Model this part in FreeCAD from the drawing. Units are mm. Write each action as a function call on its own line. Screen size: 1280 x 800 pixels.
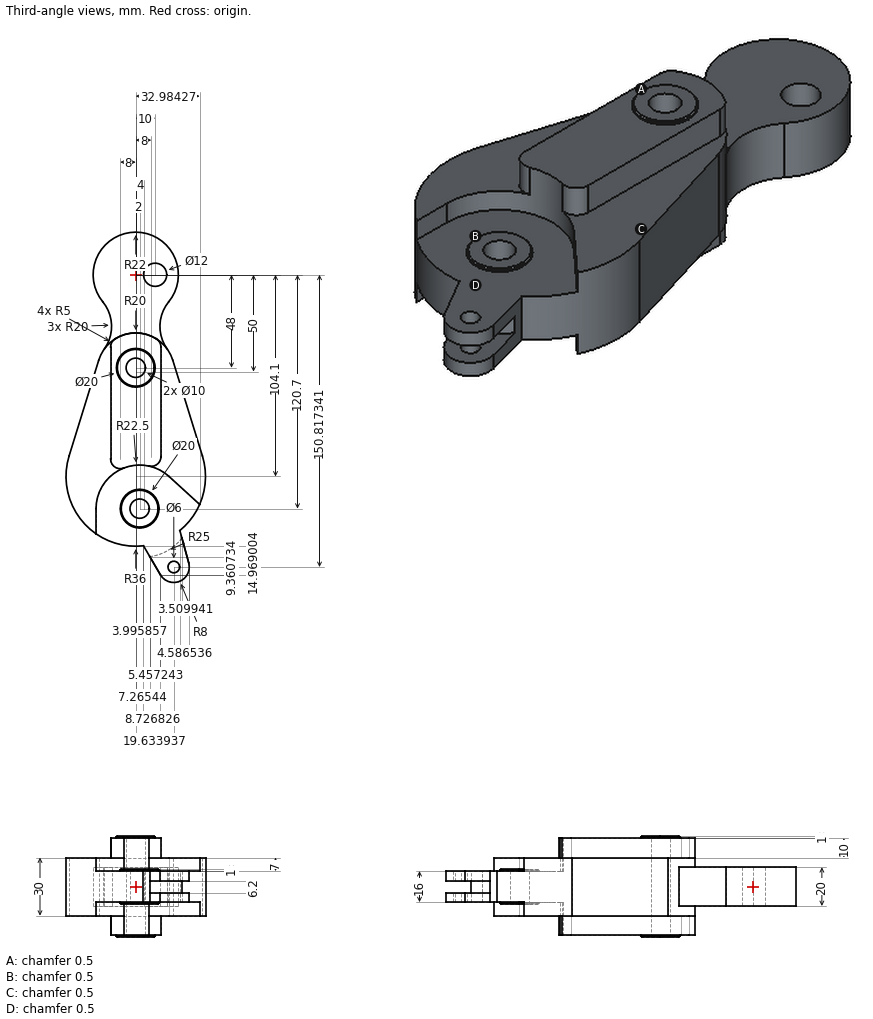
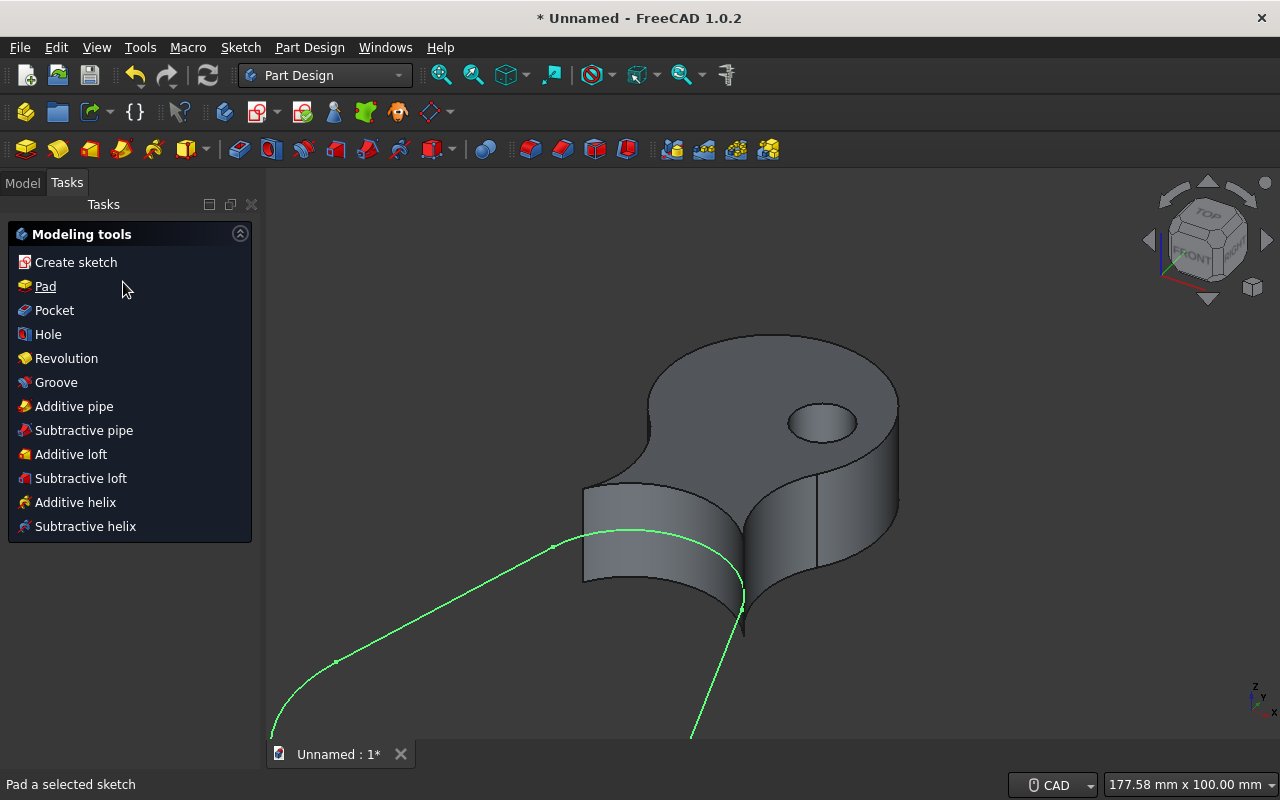
click(26, 150)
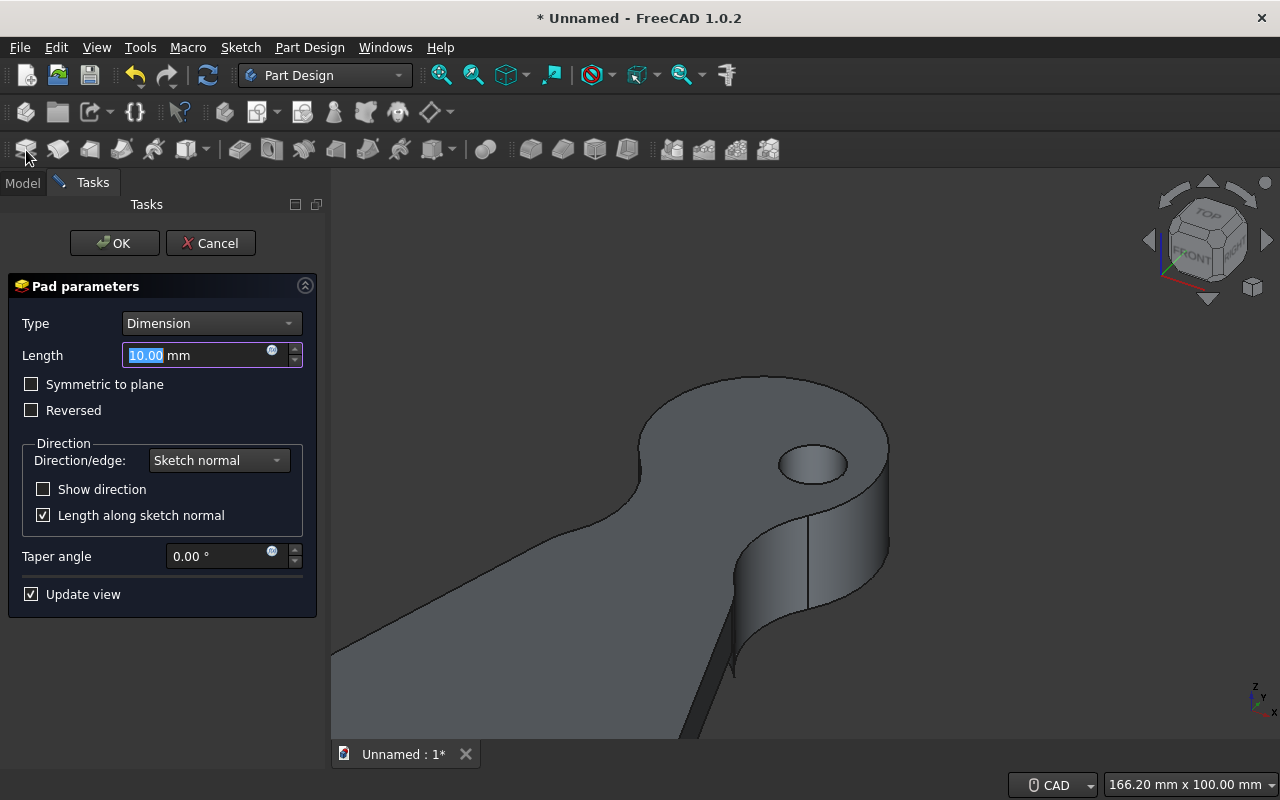
text(30)
key(Tab)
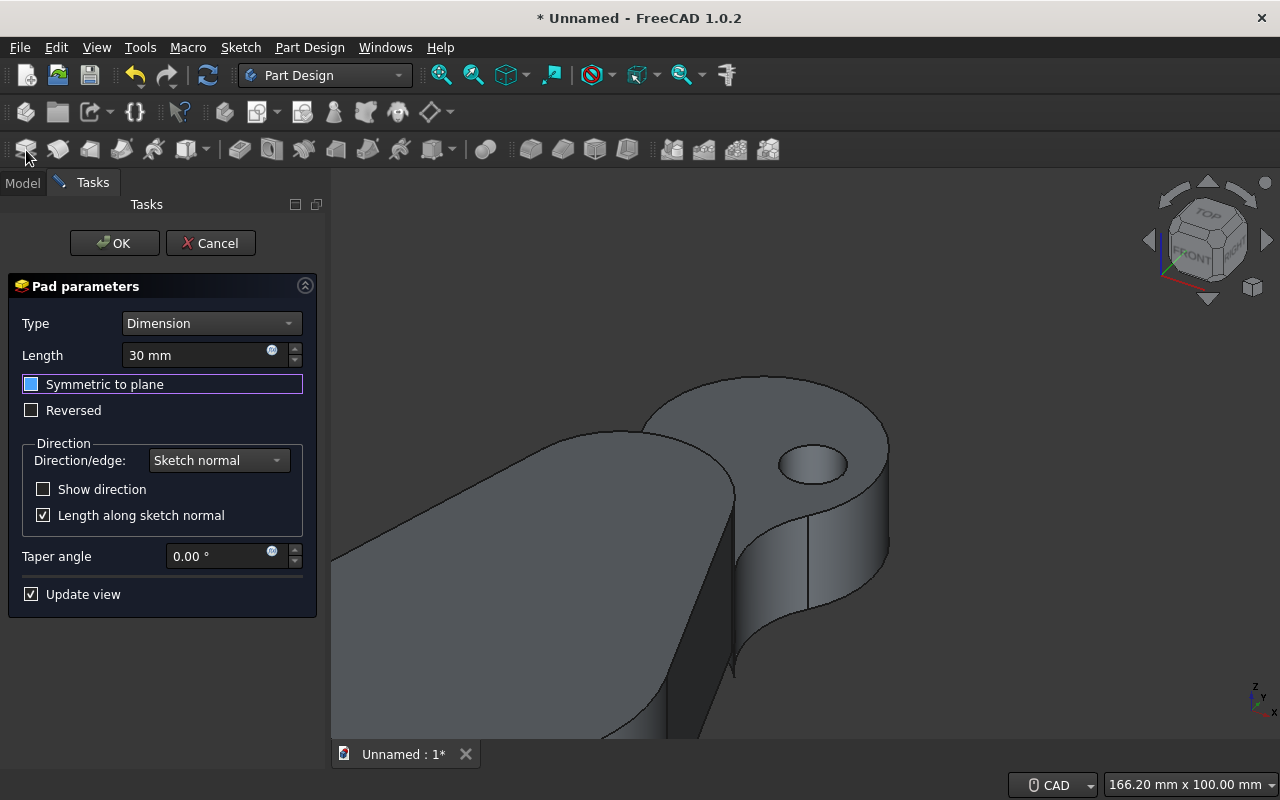
click(30, 384)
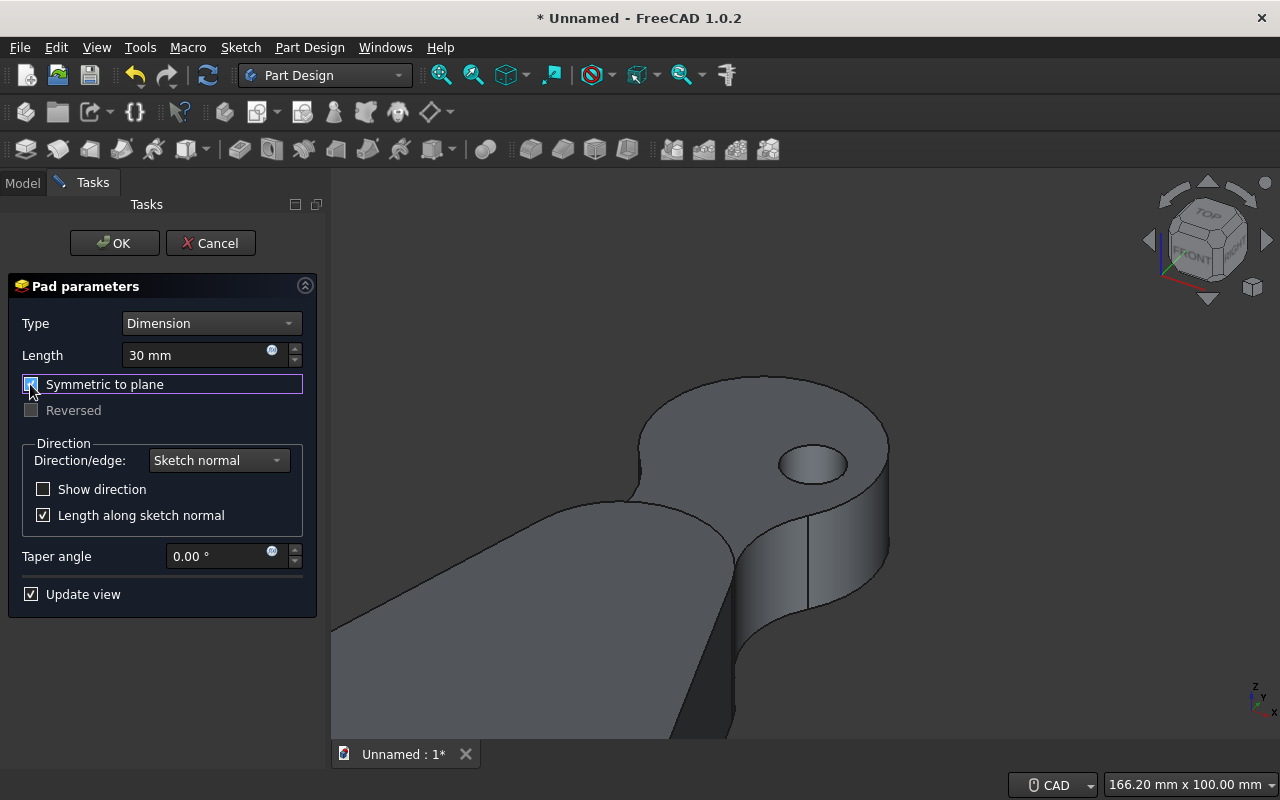
click(115, 243)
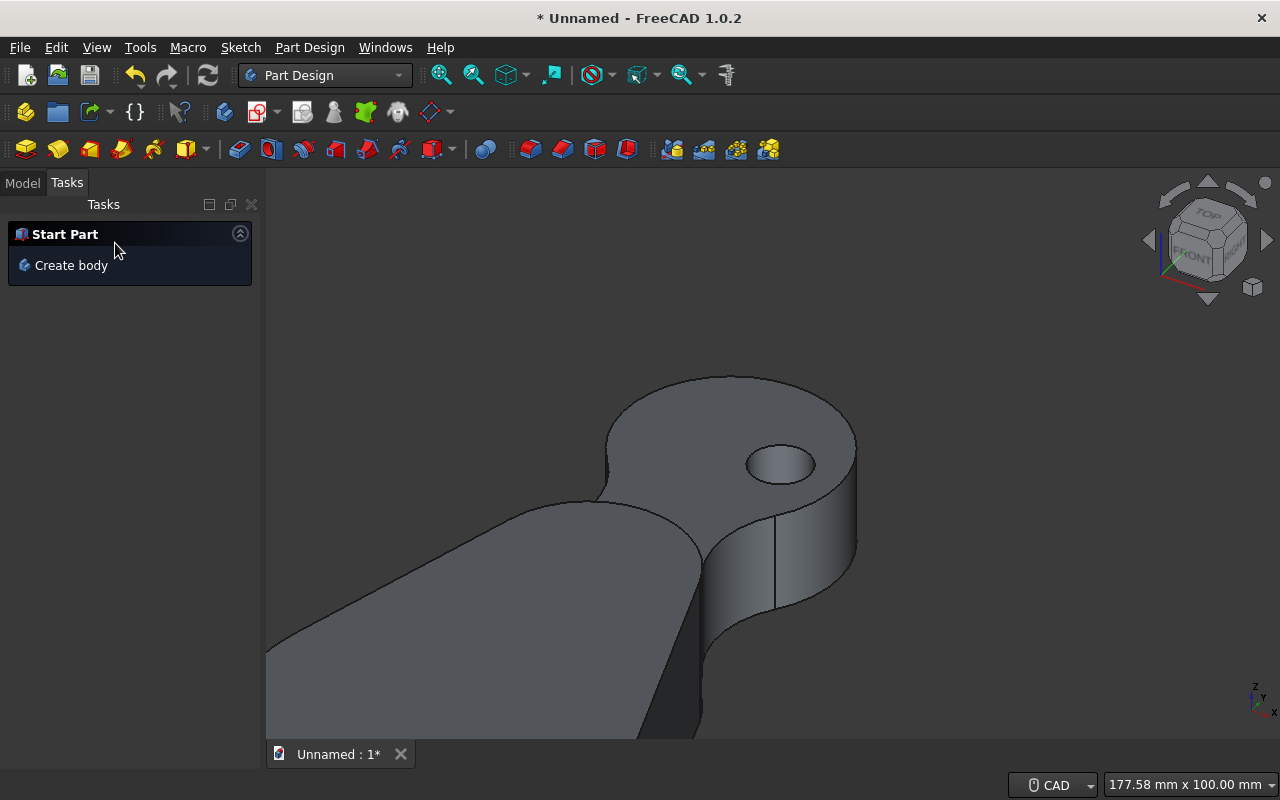
click(442, 76)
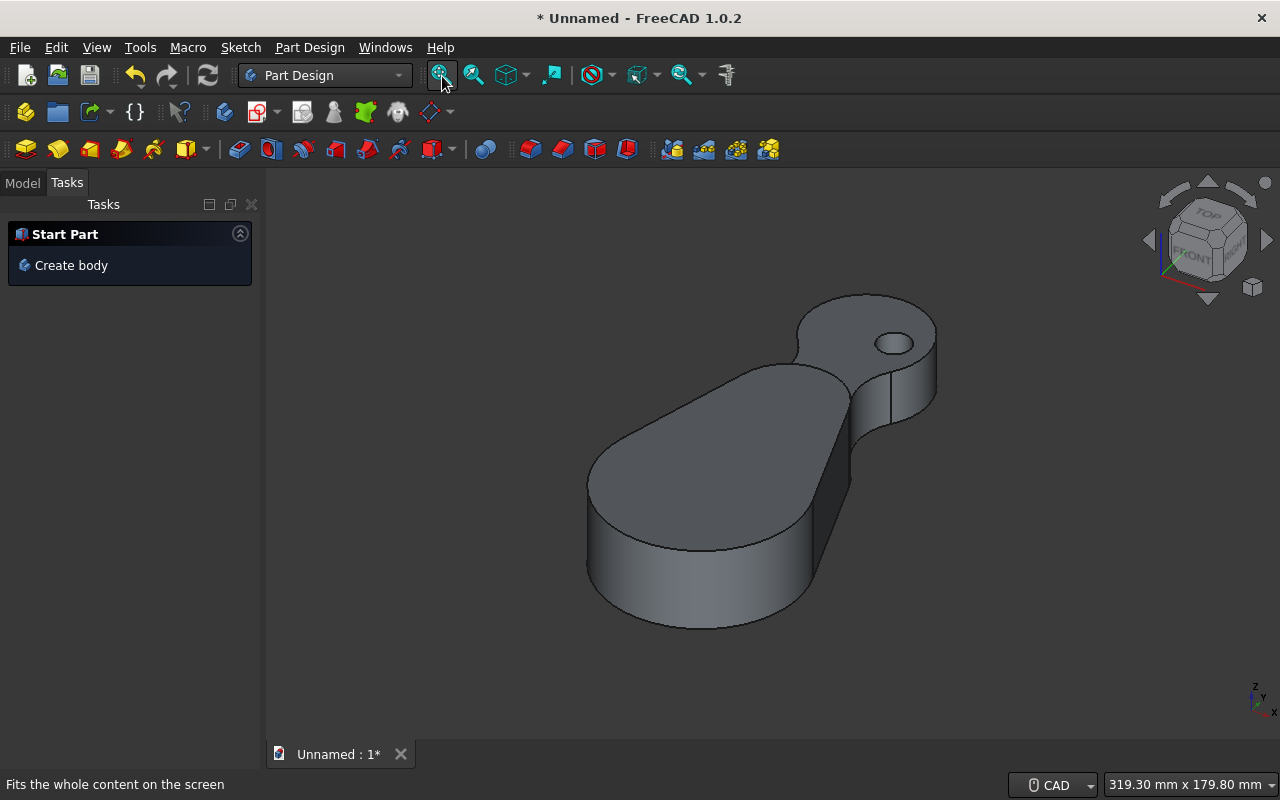
click(23, 182)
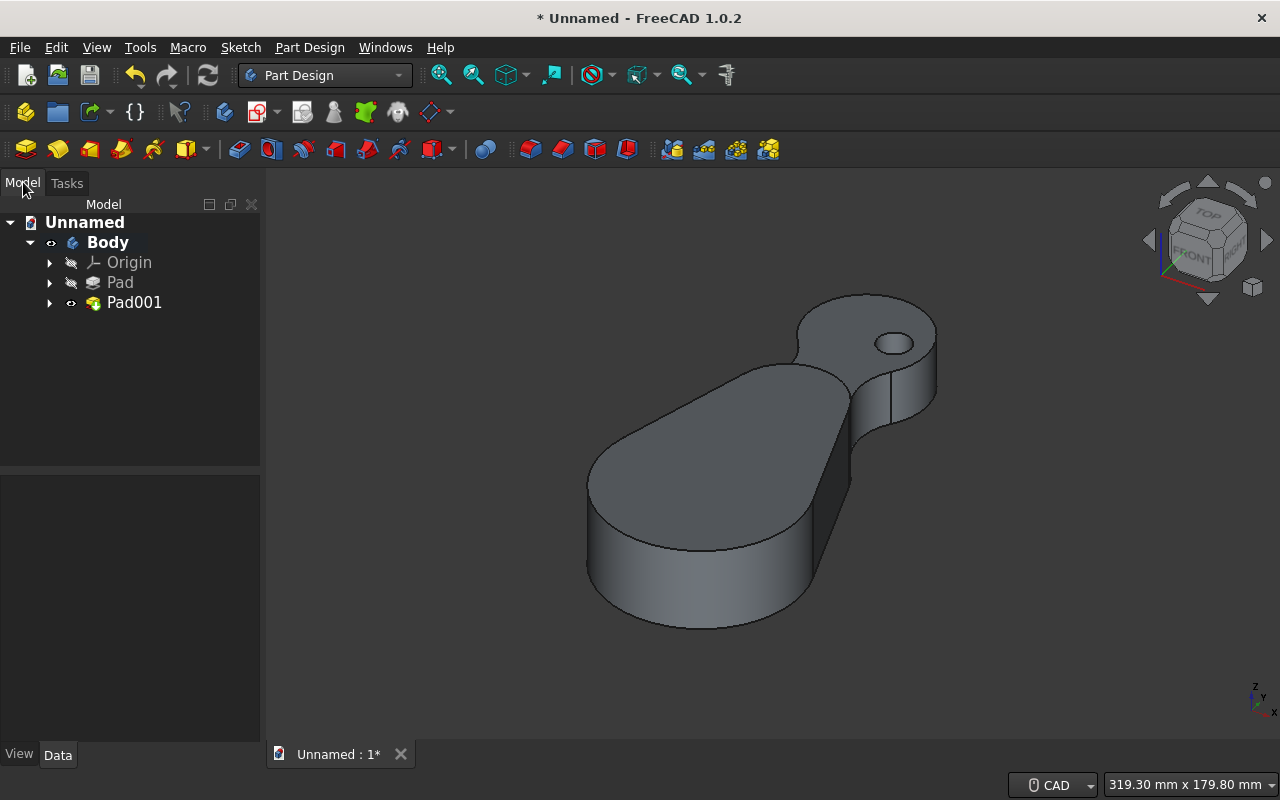
click(50, 263)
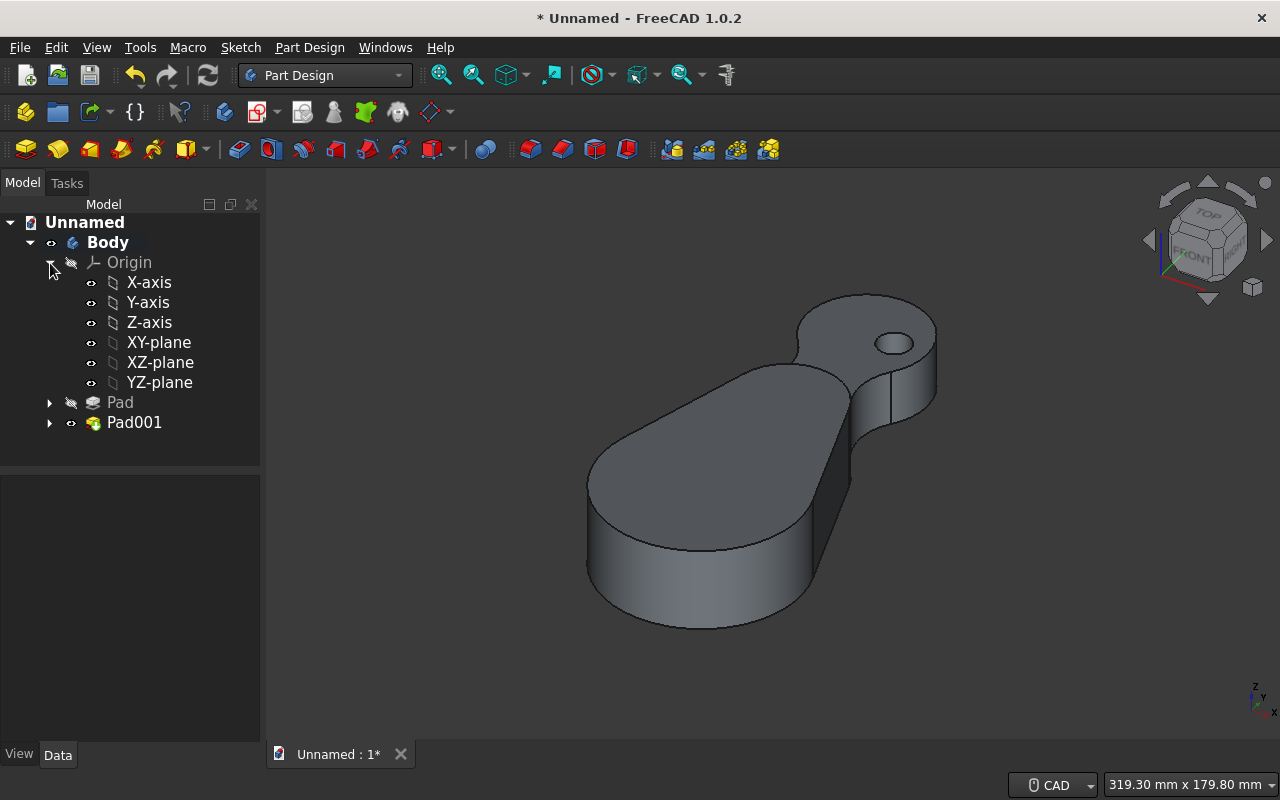
click(136, 343)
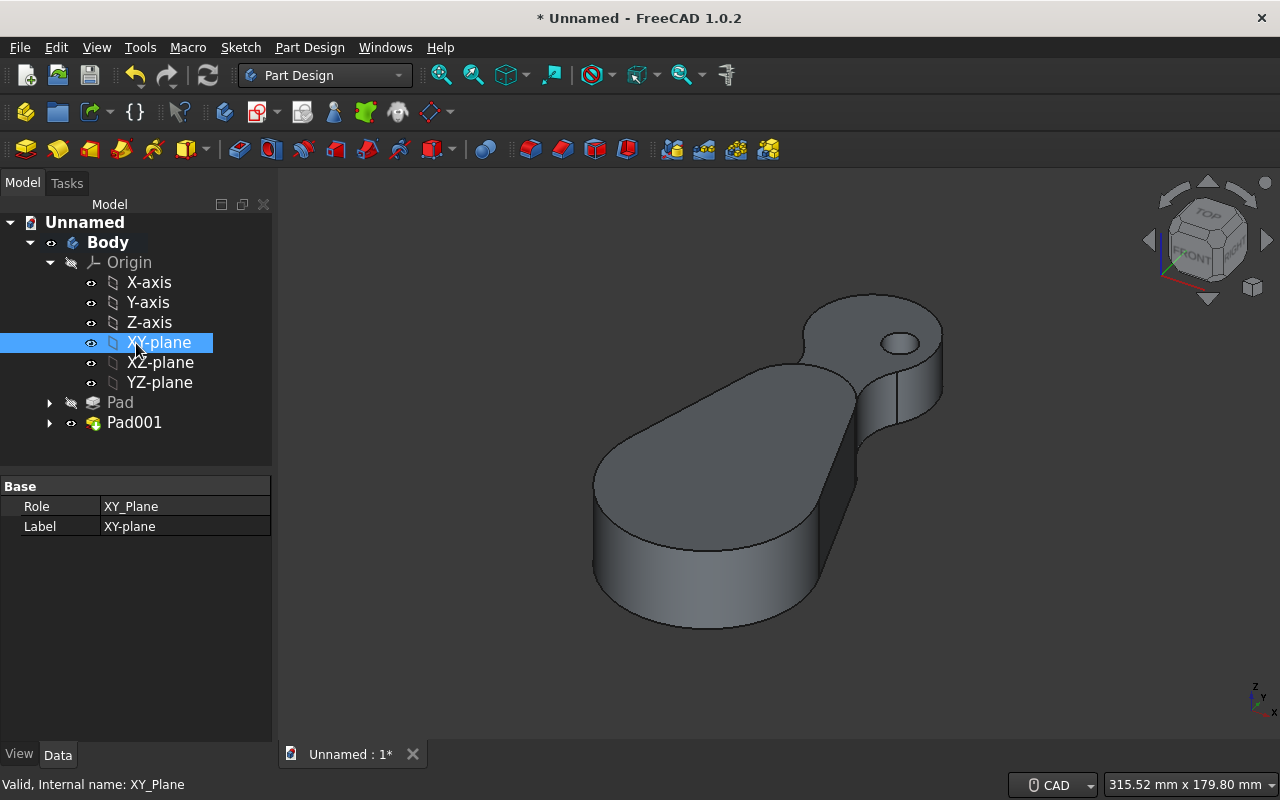
click(430, 112)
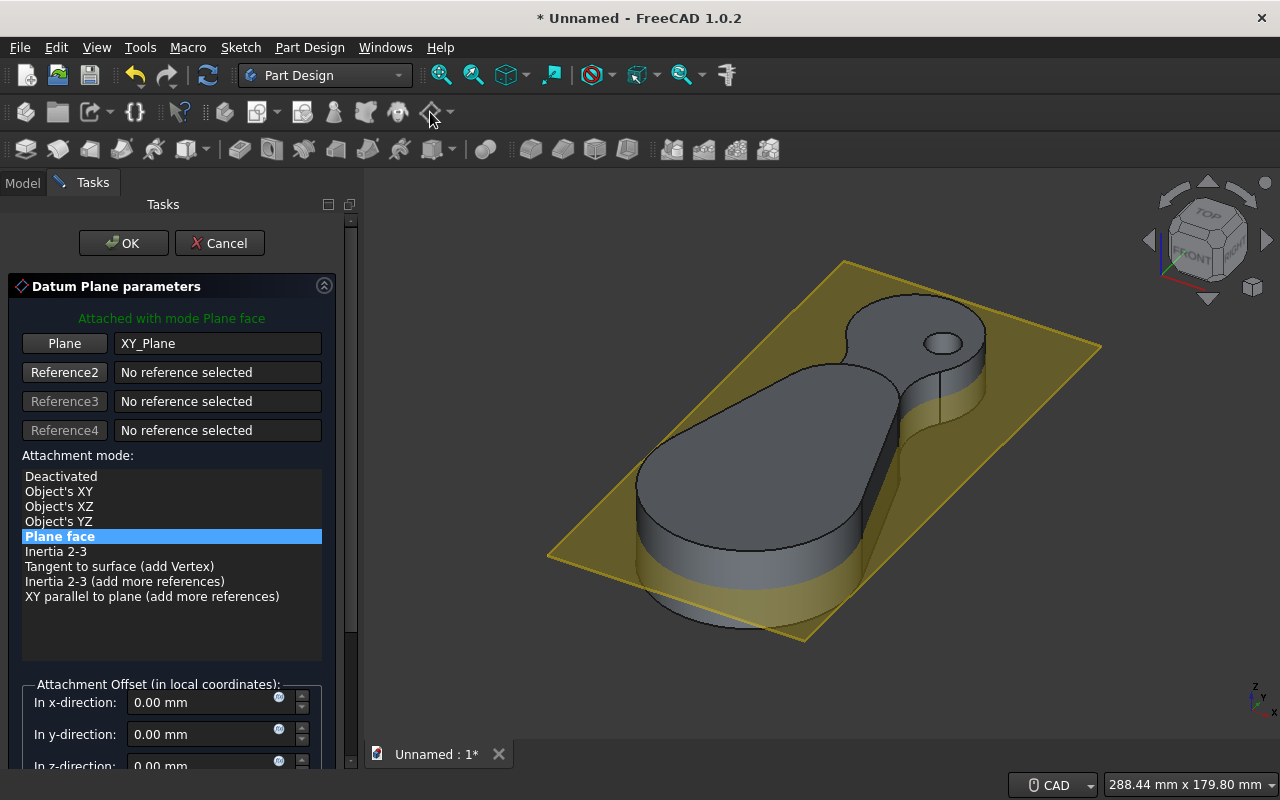
scroll(351, 491, down, 2)